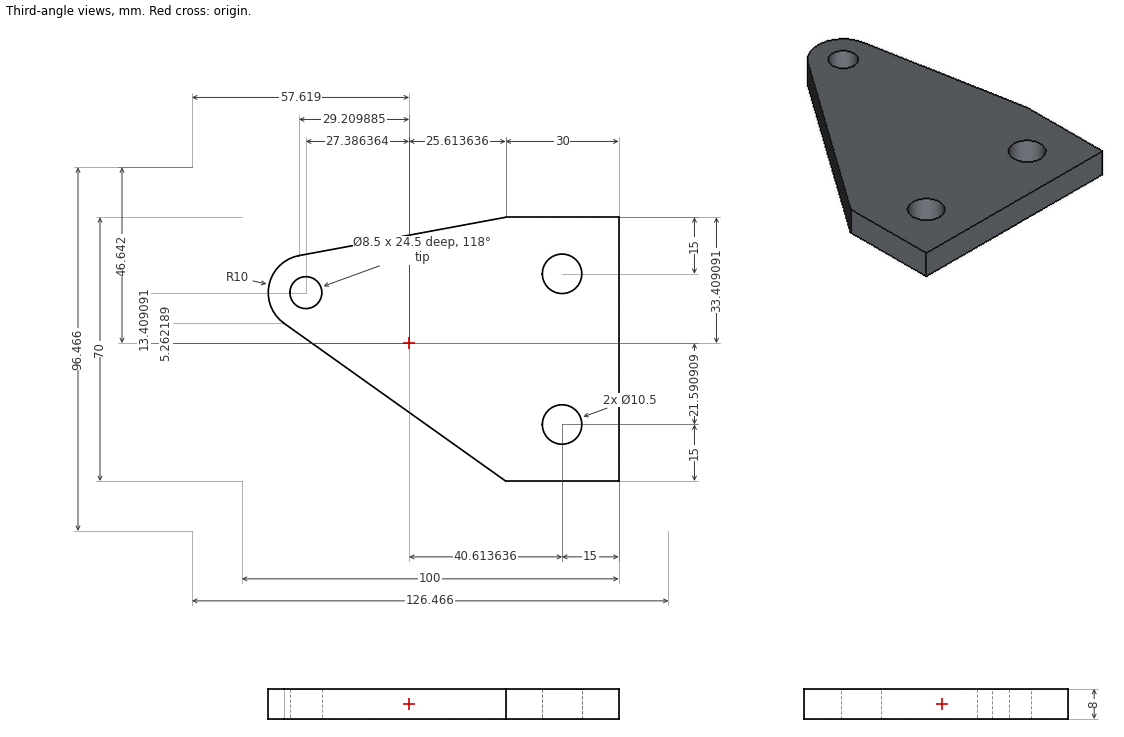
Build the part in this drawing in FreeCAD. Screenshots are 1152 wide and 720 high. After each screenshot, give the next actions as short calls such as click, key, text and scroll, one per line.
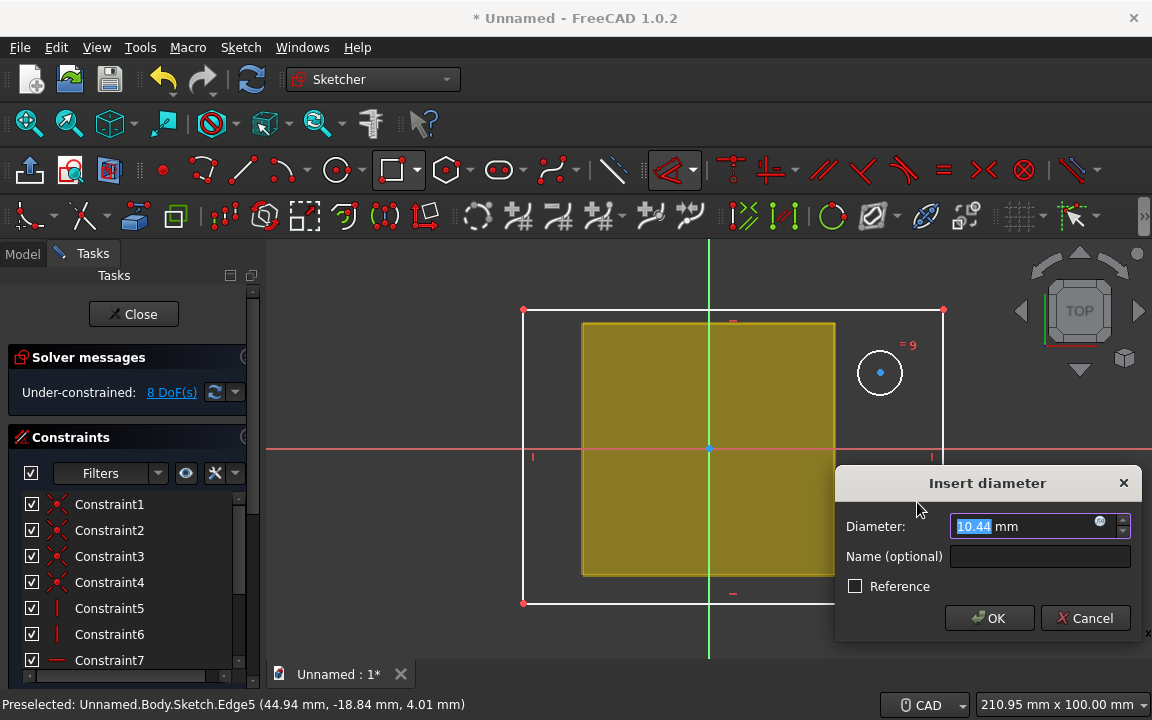
text(10.5)
key(Return)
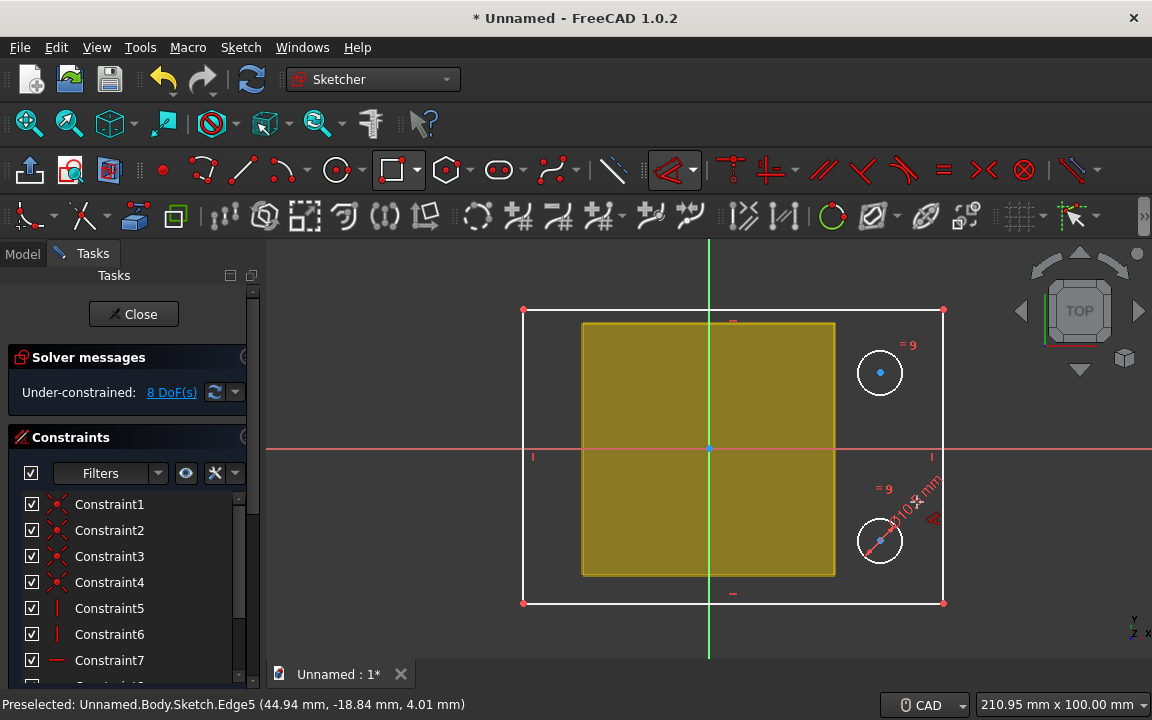
click(523, 398)
click(489, 389)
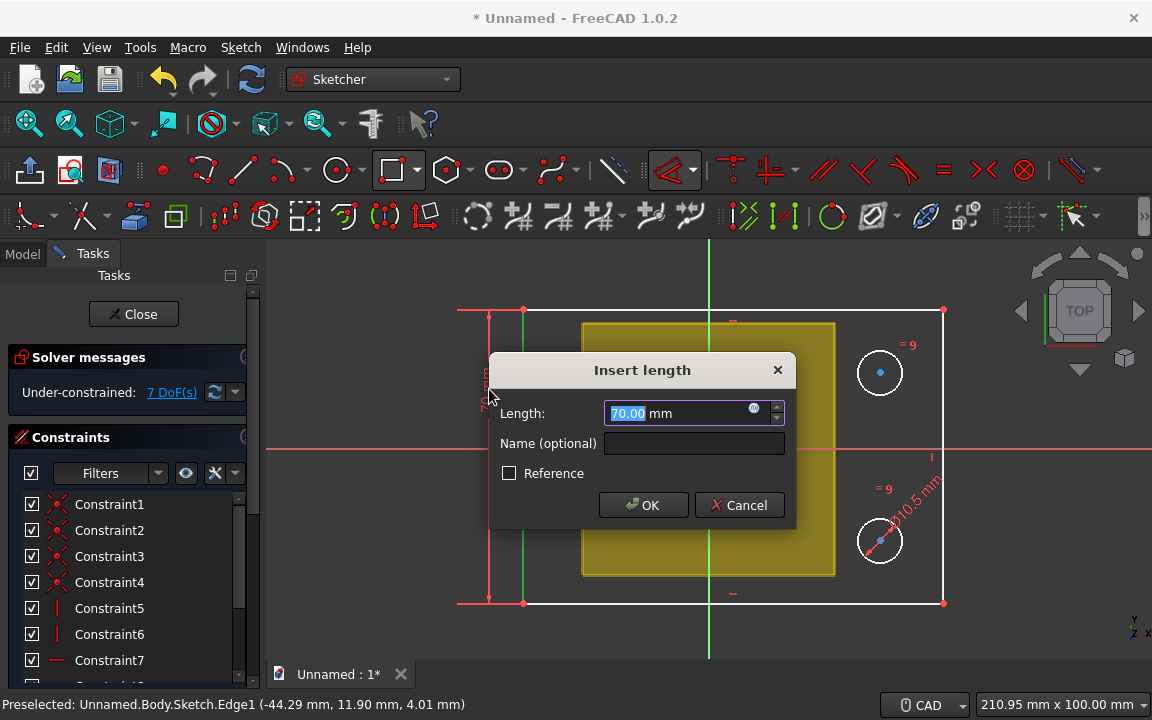
text(70)
key(Return)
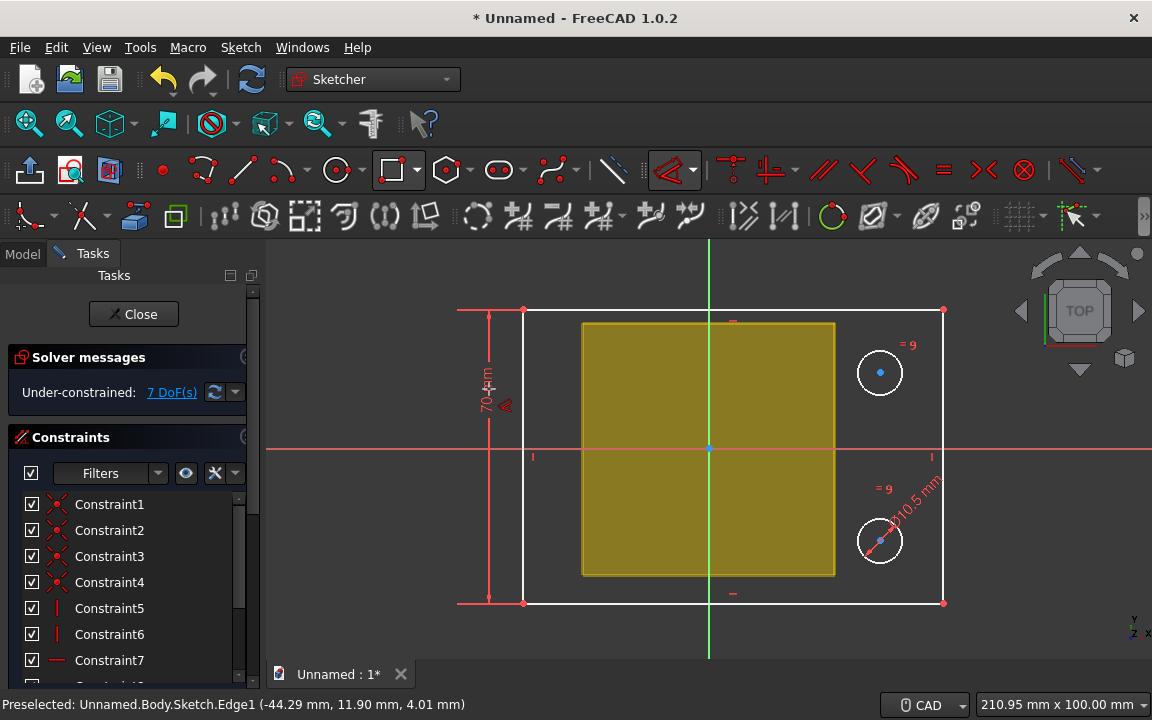
click(649, 604)
click(733, 570)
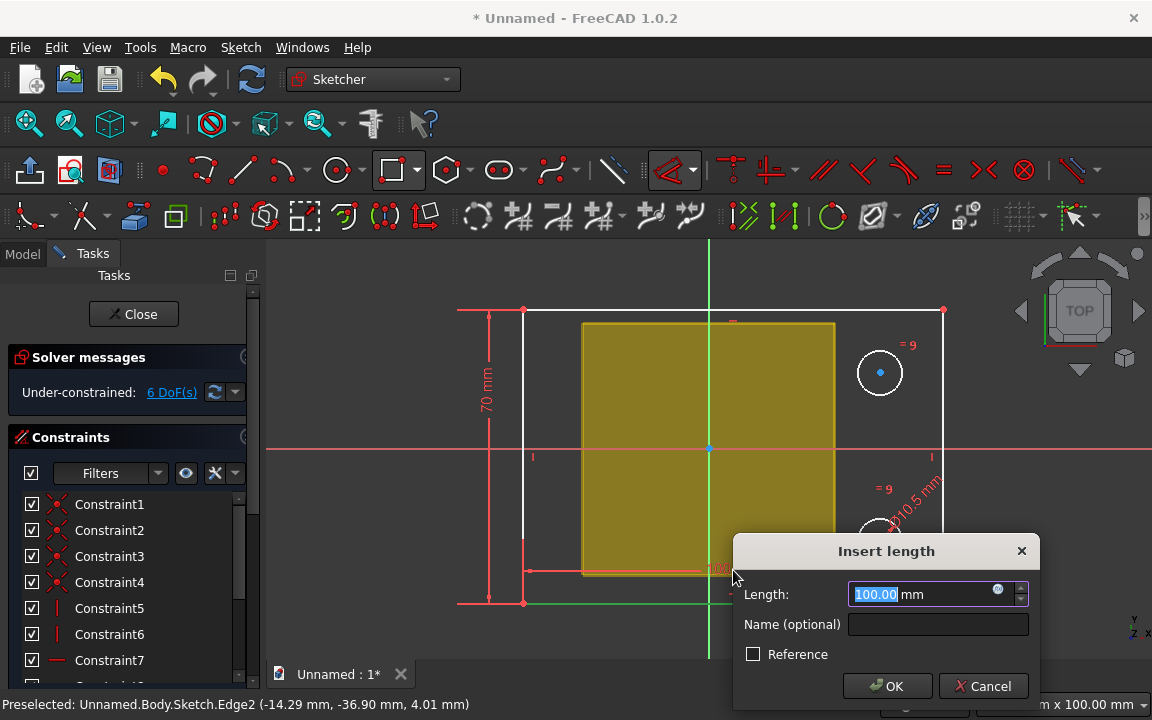
text(100)
key(Return)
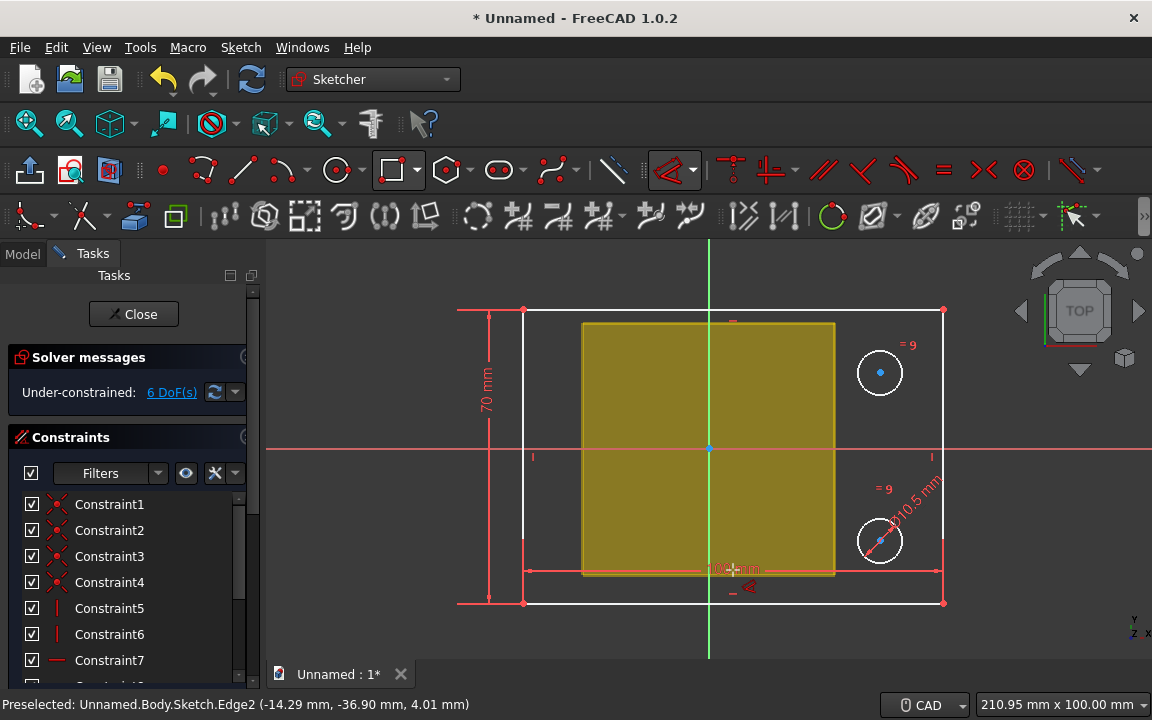
click(943, 604)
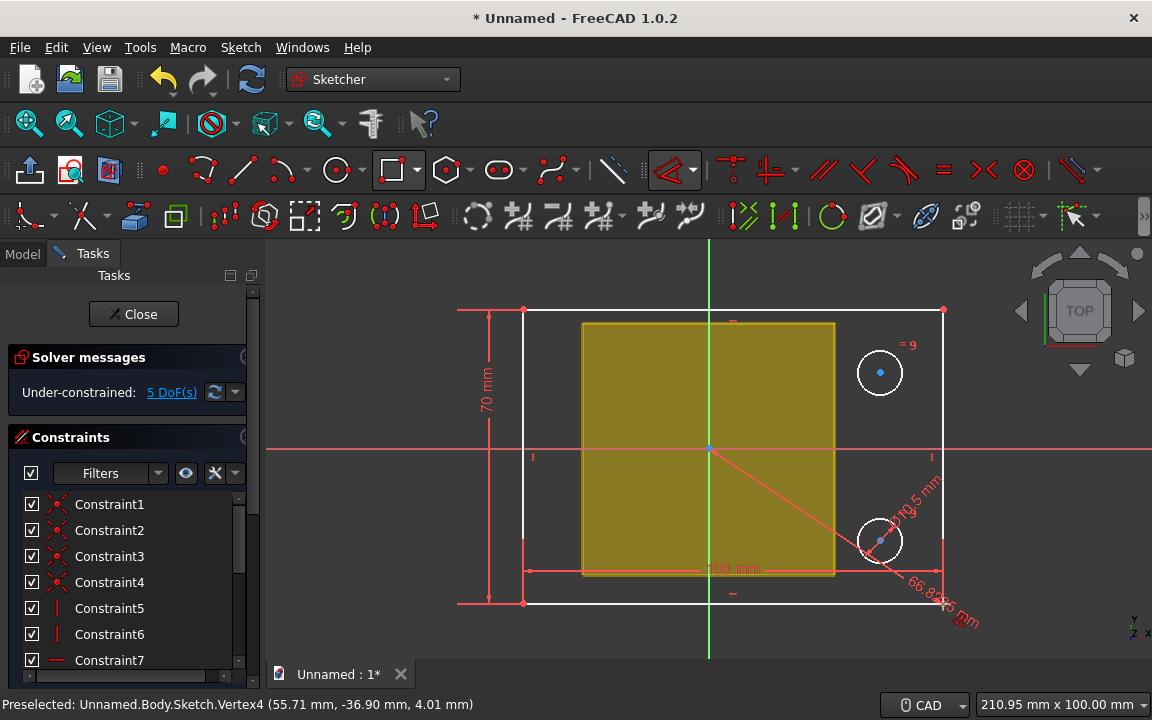
click(880, 541)
click(912, 435)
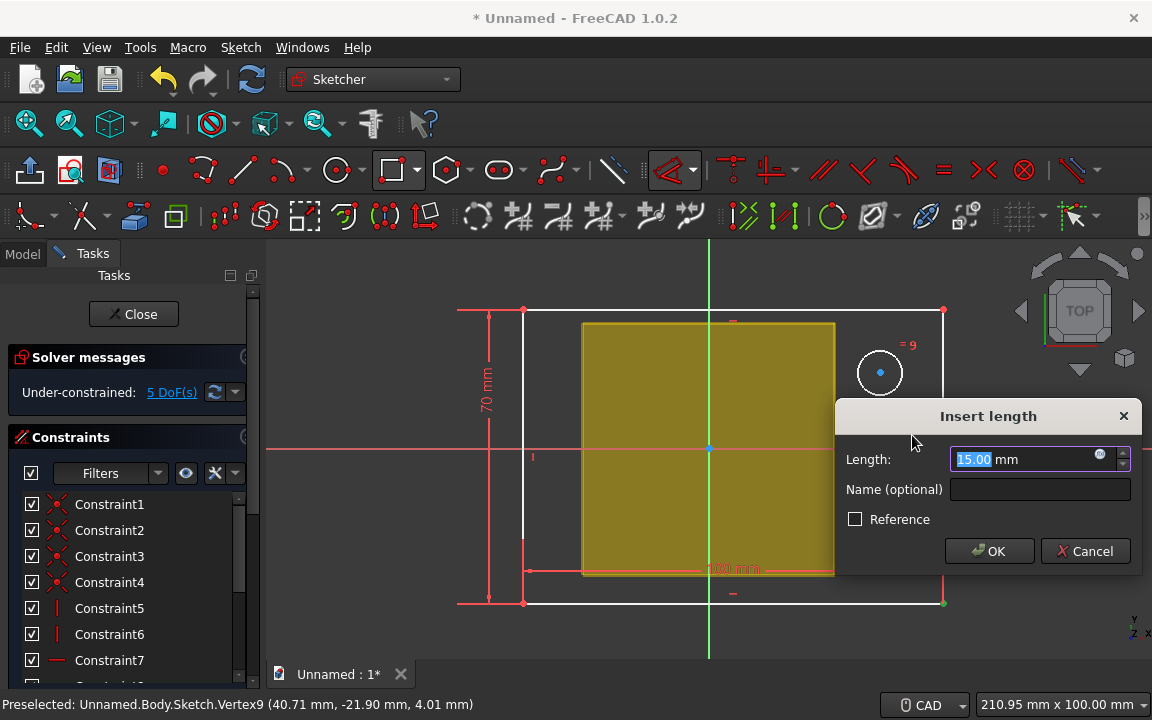
text(15)
key(Return)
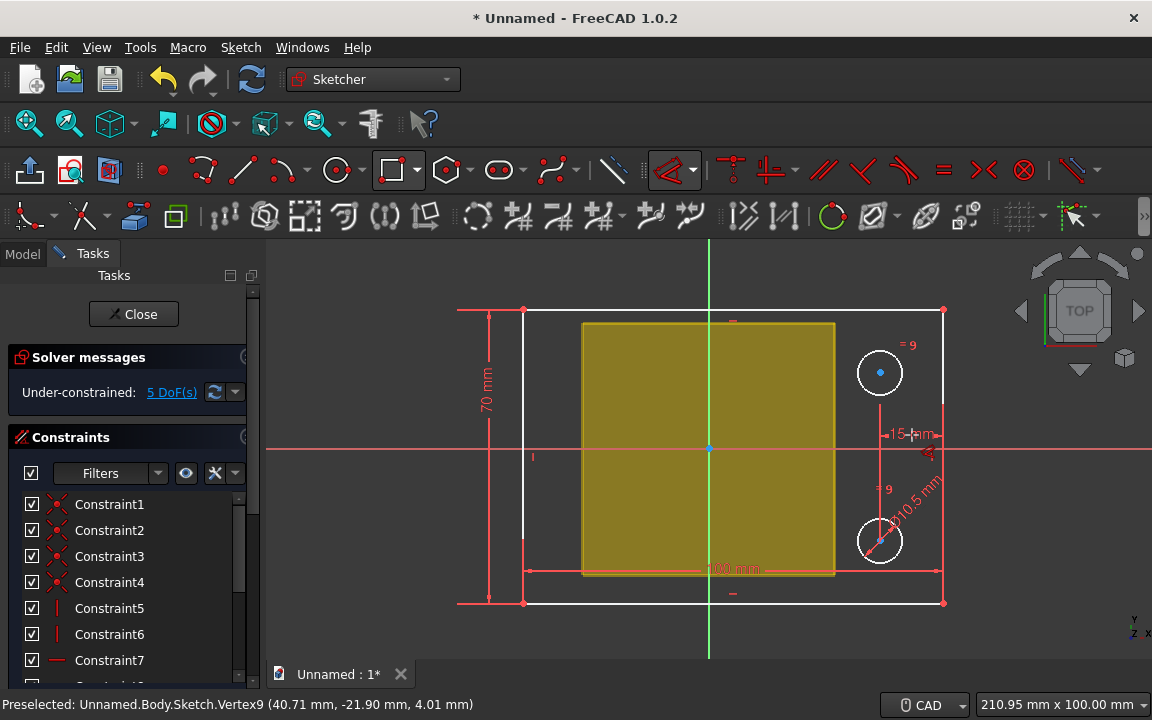
click(943, 604)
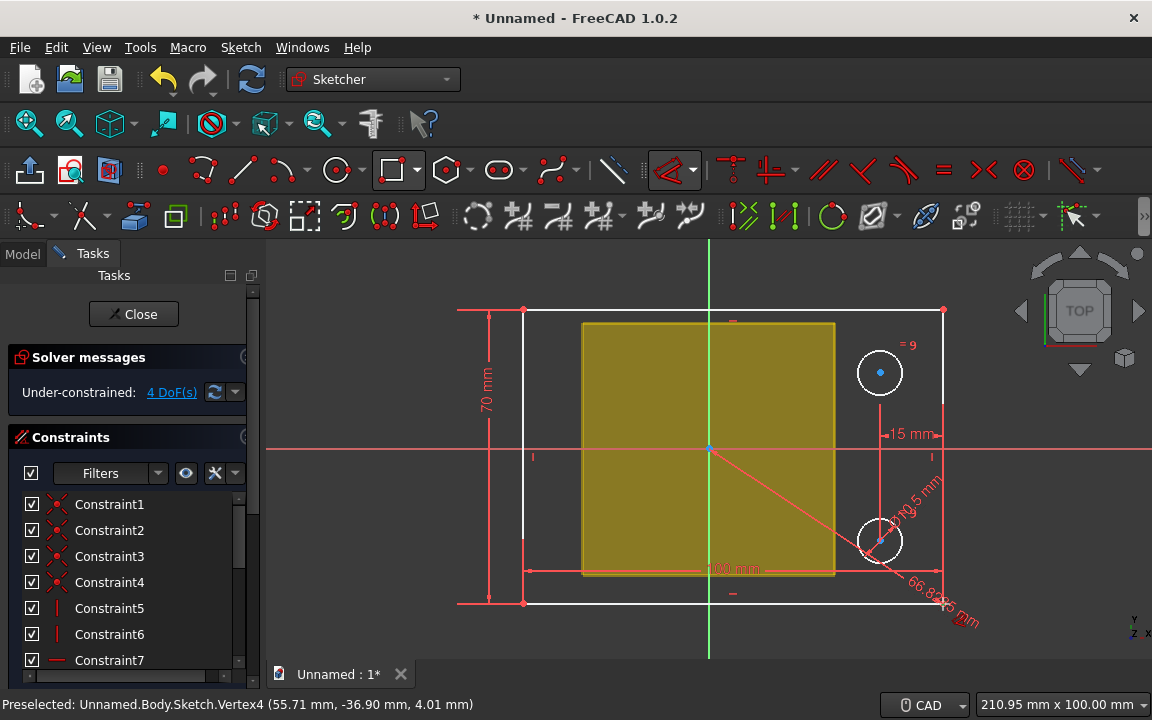
click(880, 541)
click(977, 572)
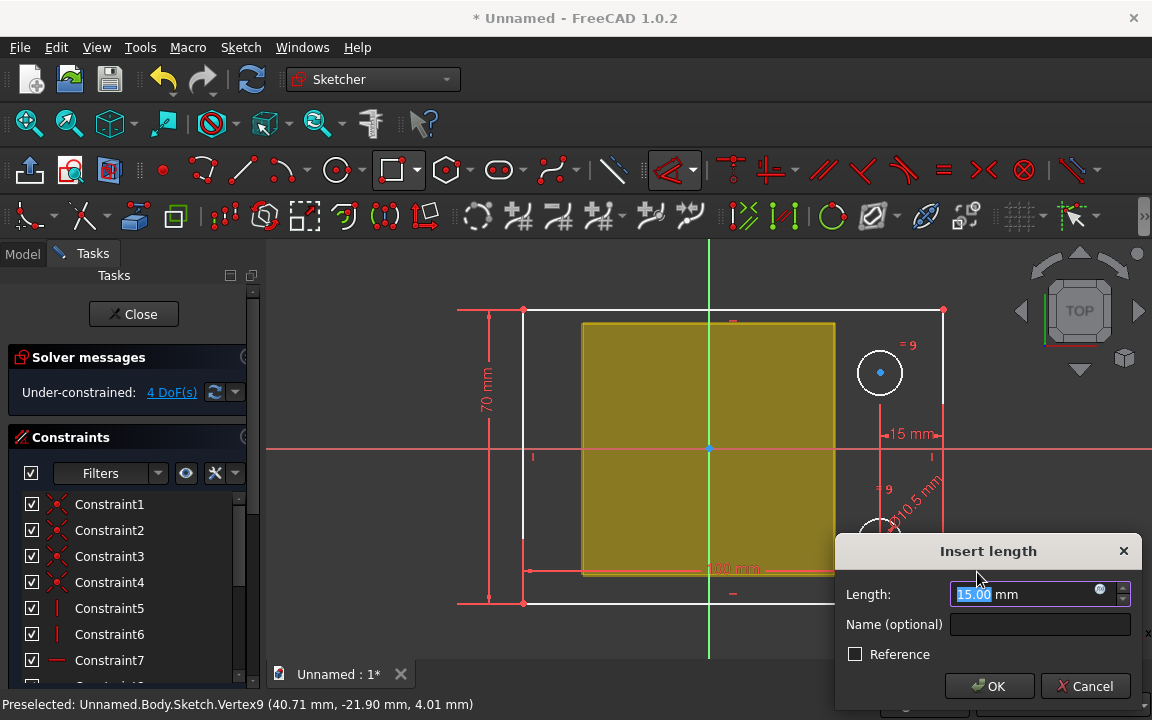
text(15)
key(Return)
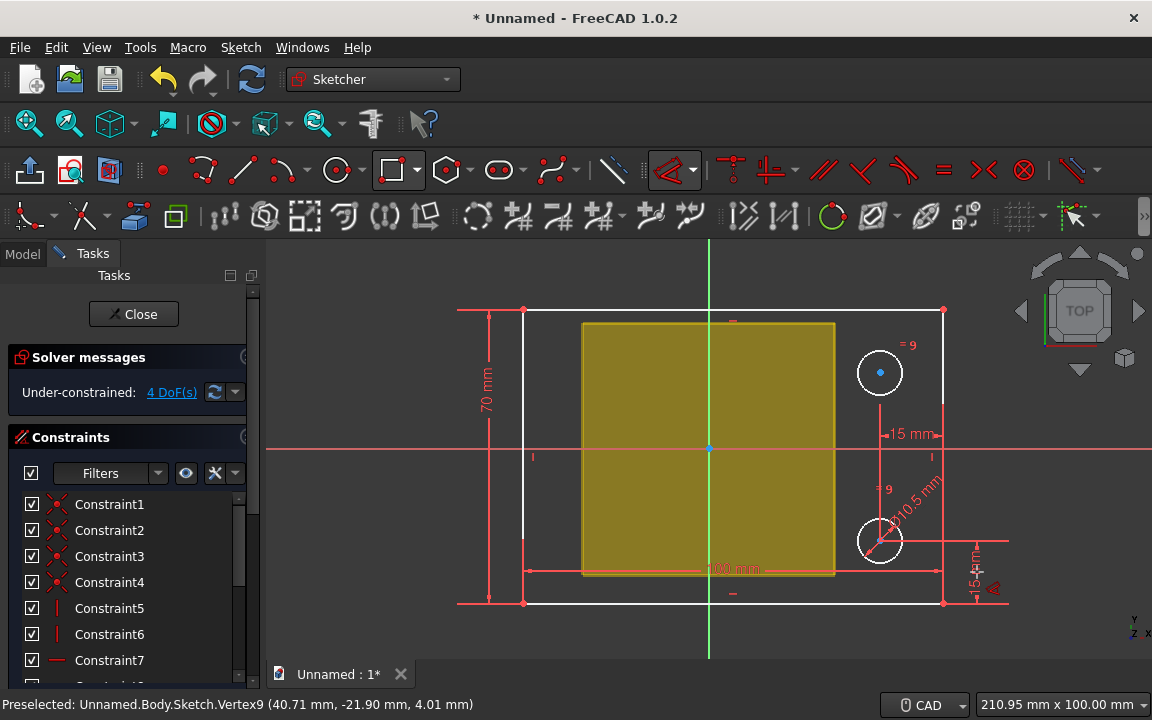
click(943, 310)